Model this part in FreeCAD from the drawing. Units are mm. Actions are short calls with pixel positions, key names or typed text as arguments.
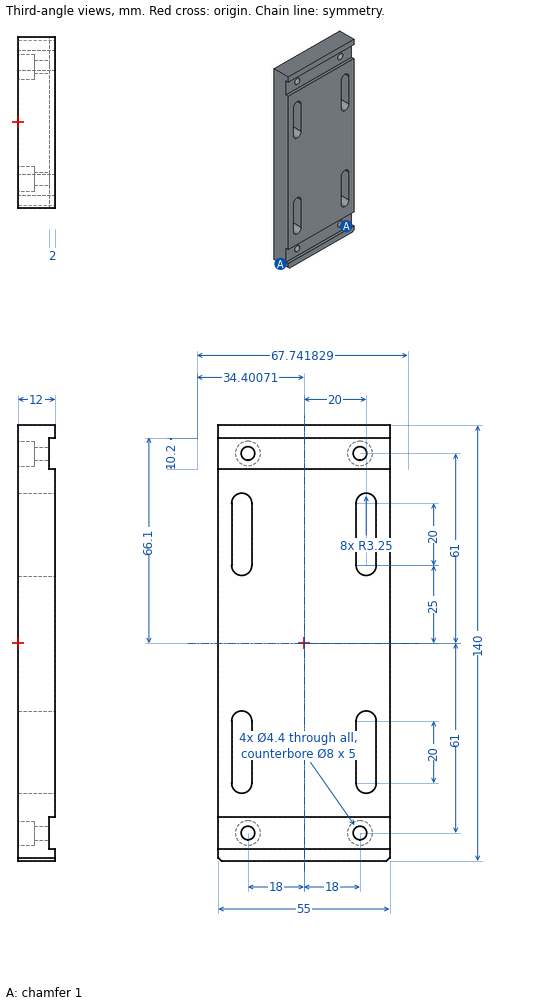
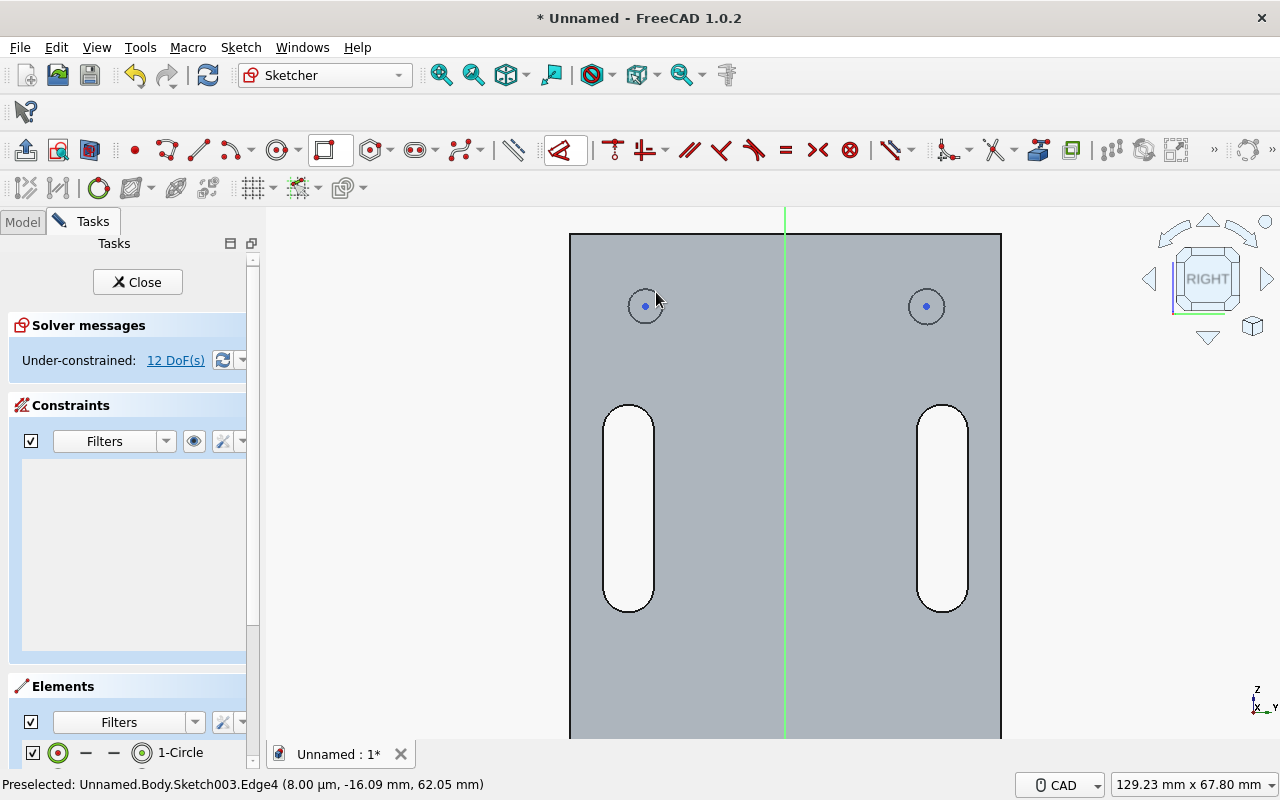
scroll(657, 292, down, 5)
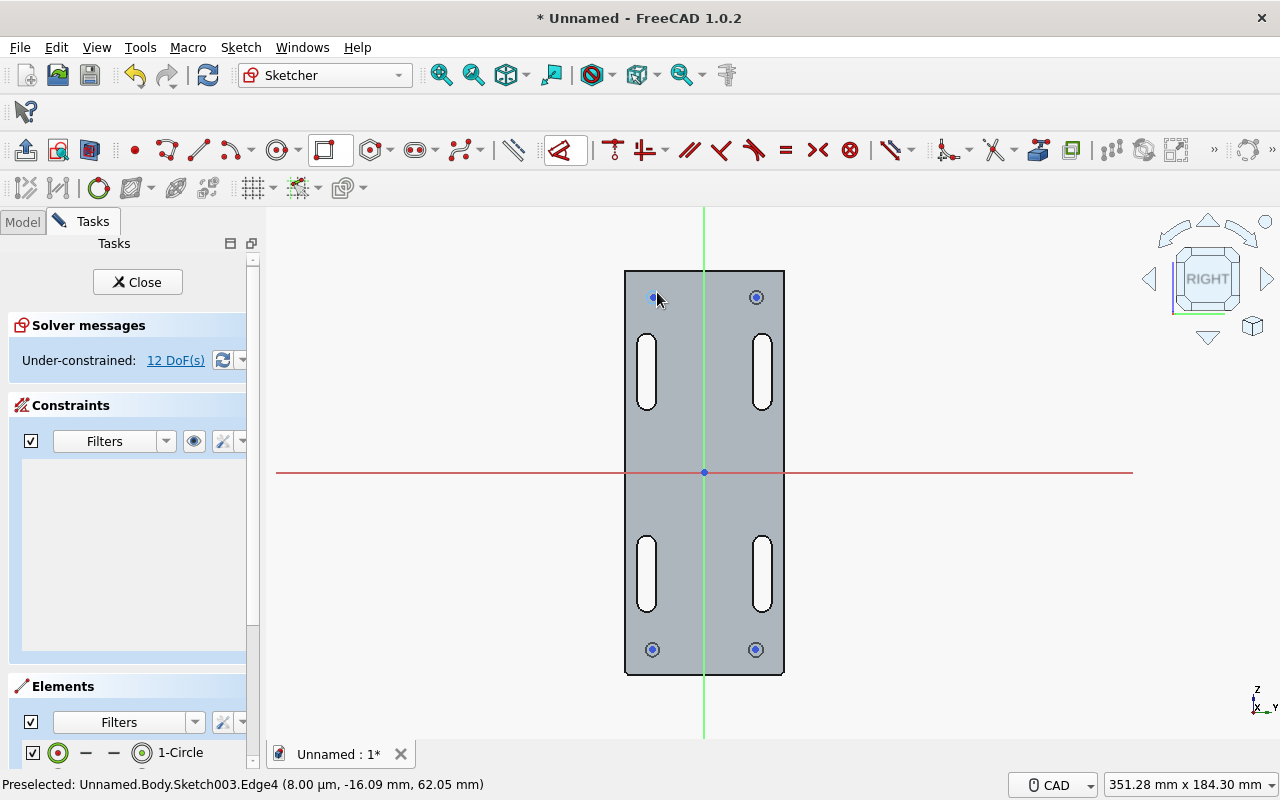
scroll(761, 645, up, 4)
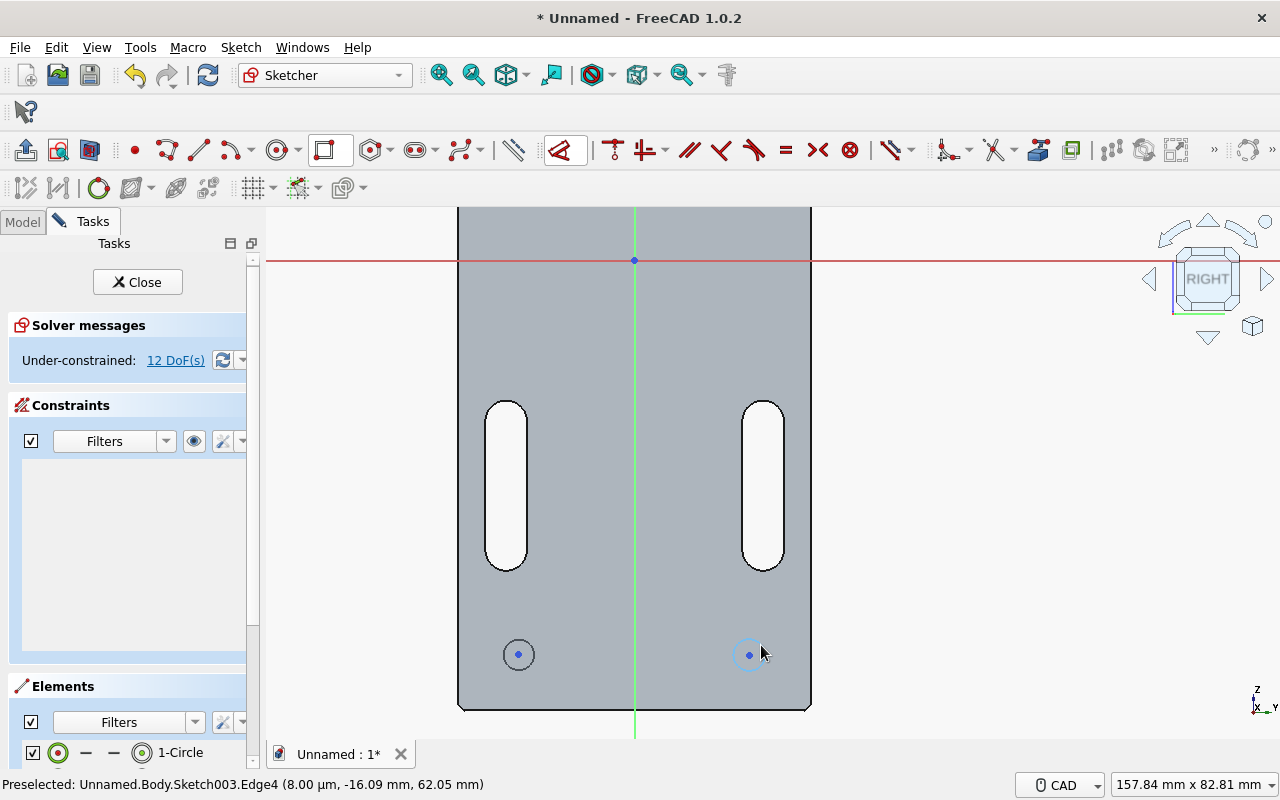
click(760, 644)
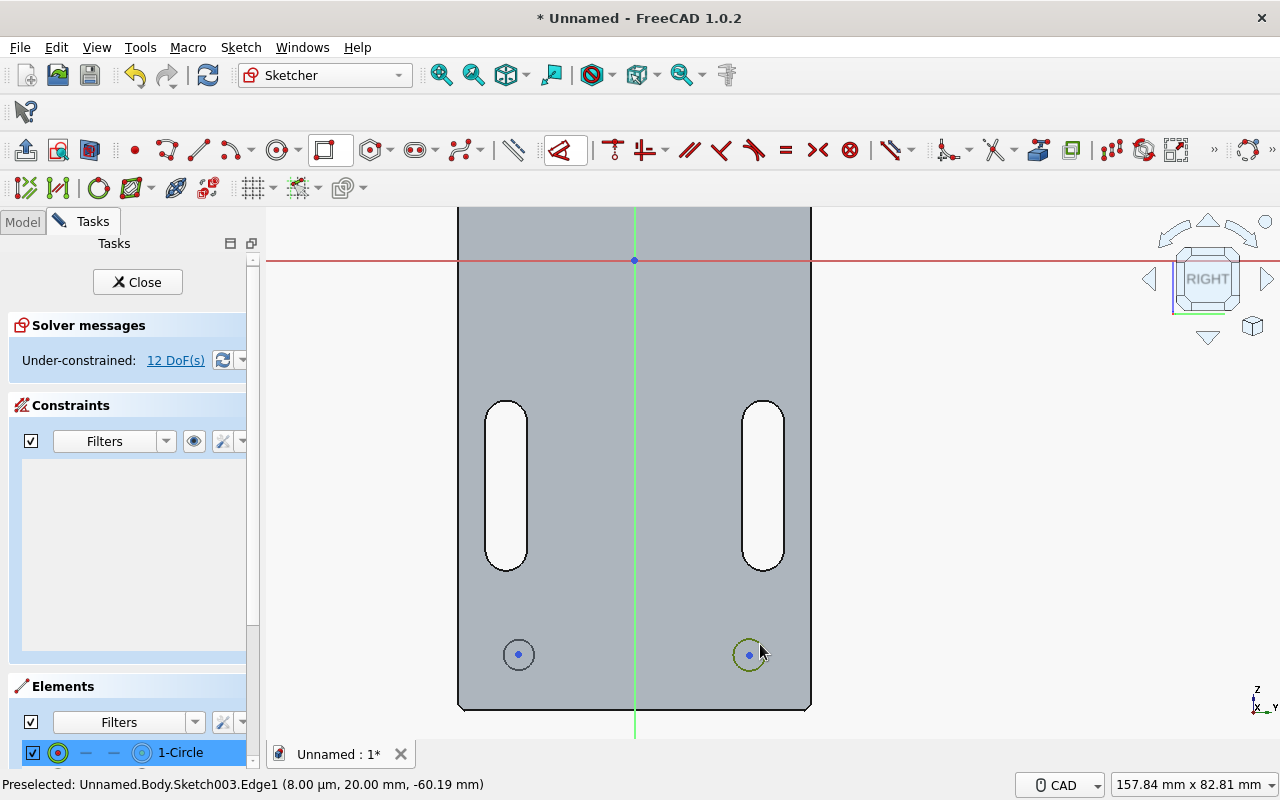
click(530, 644)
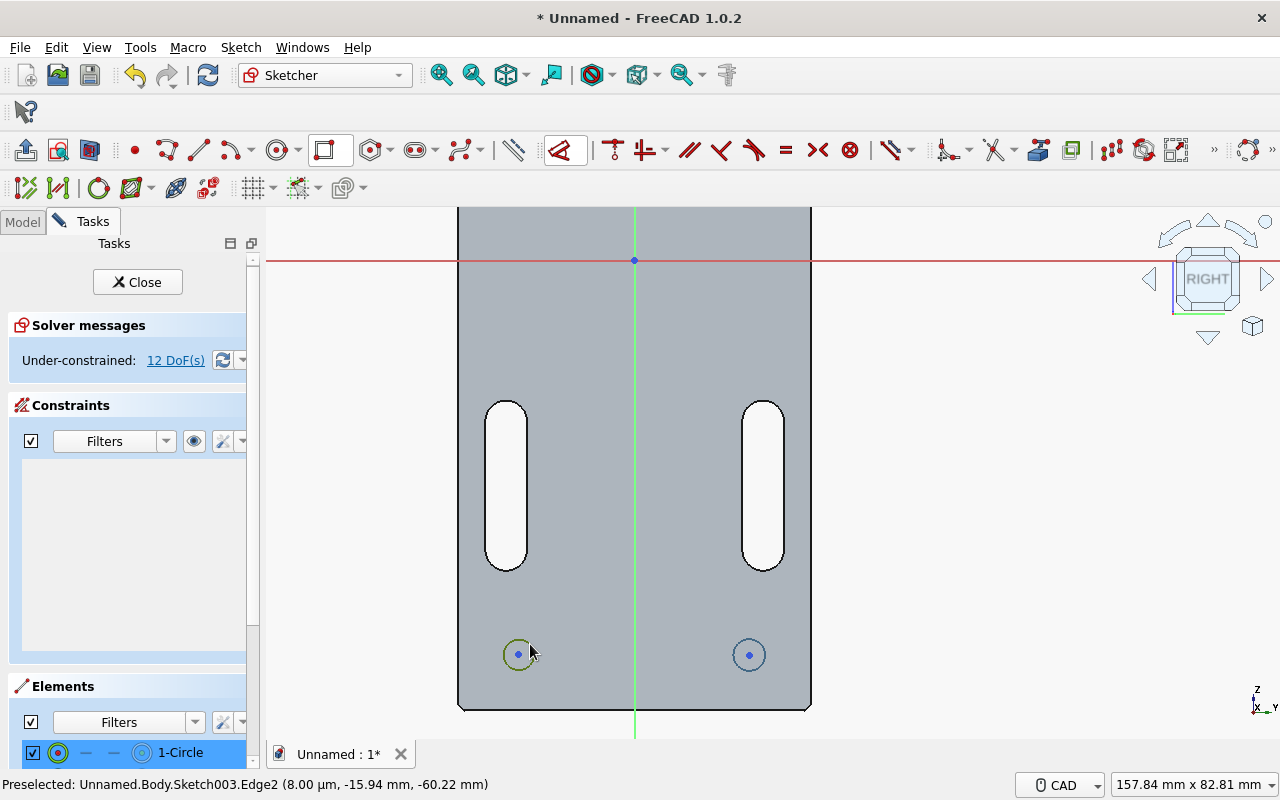
scroll(762, 646, down, 4)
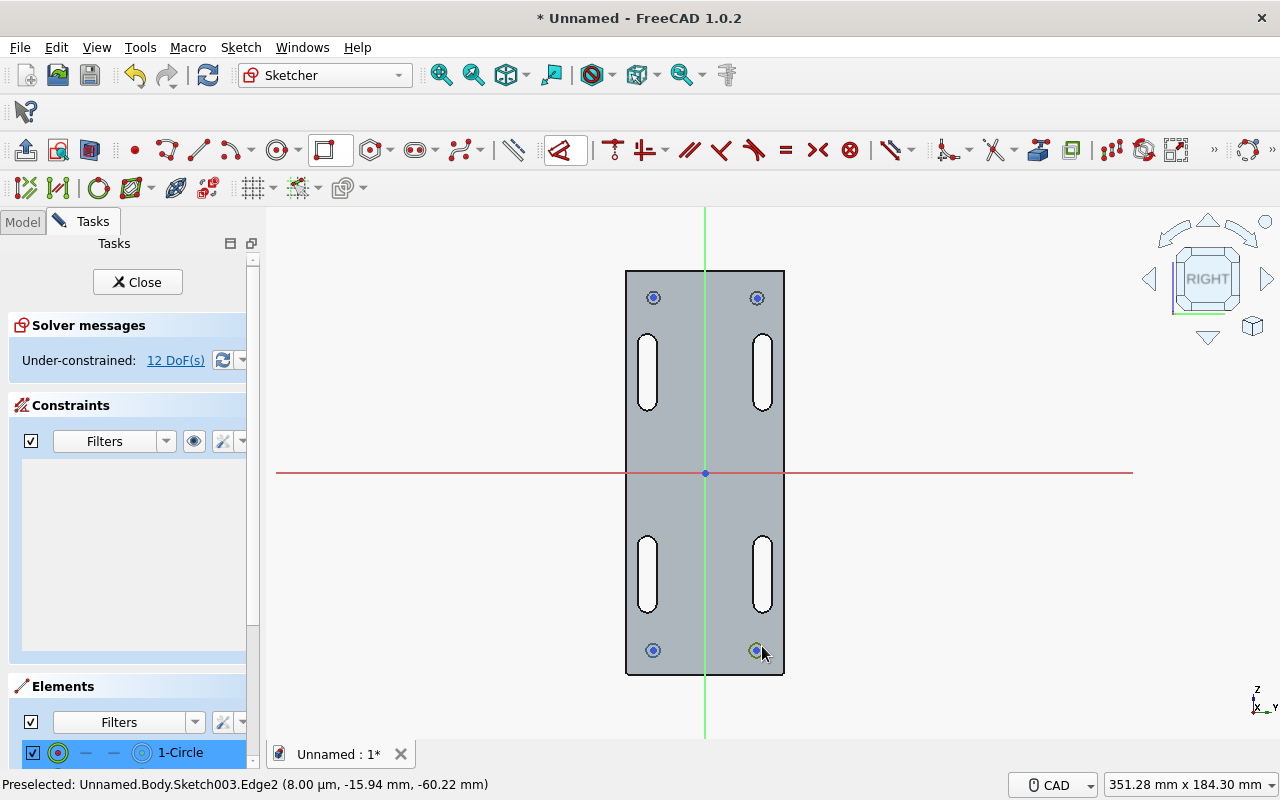
scroll(762, 293, up, 4)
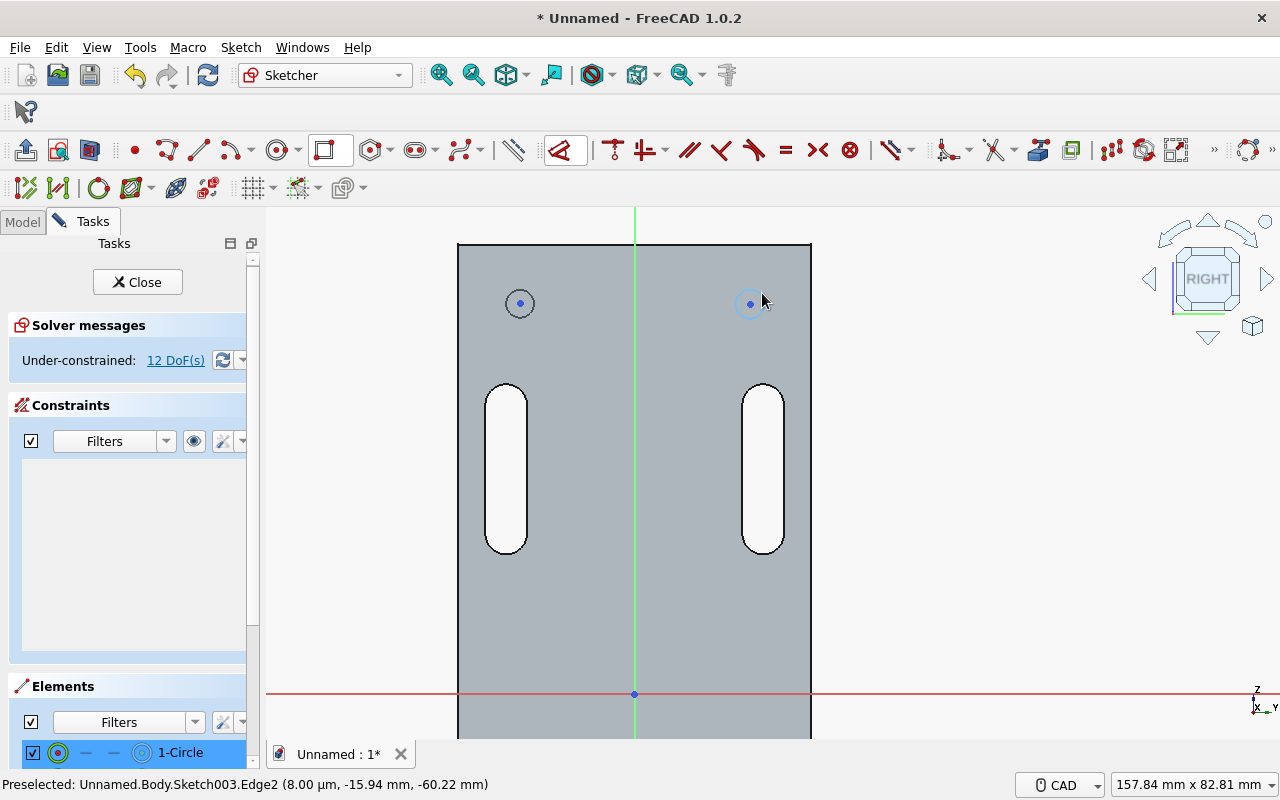
click(761, 294)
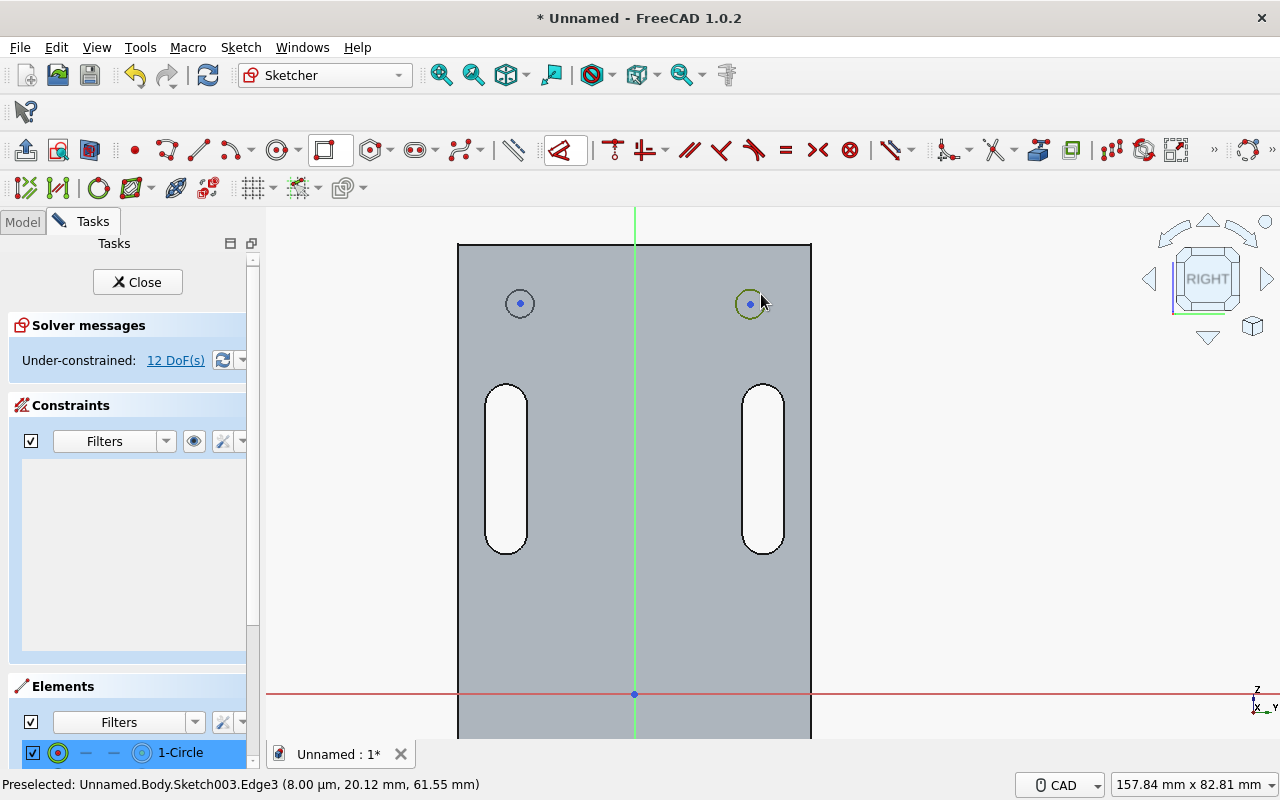
click(530, 294)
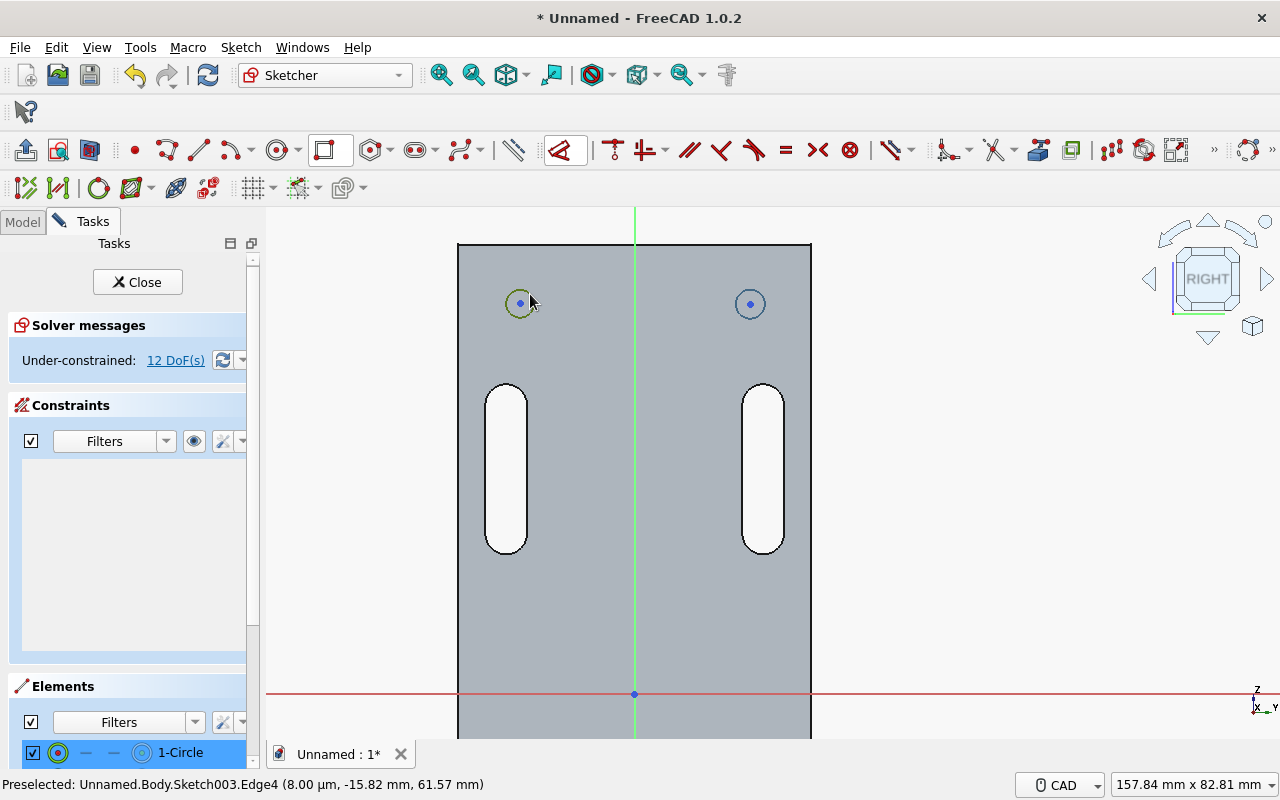
click(786, 150)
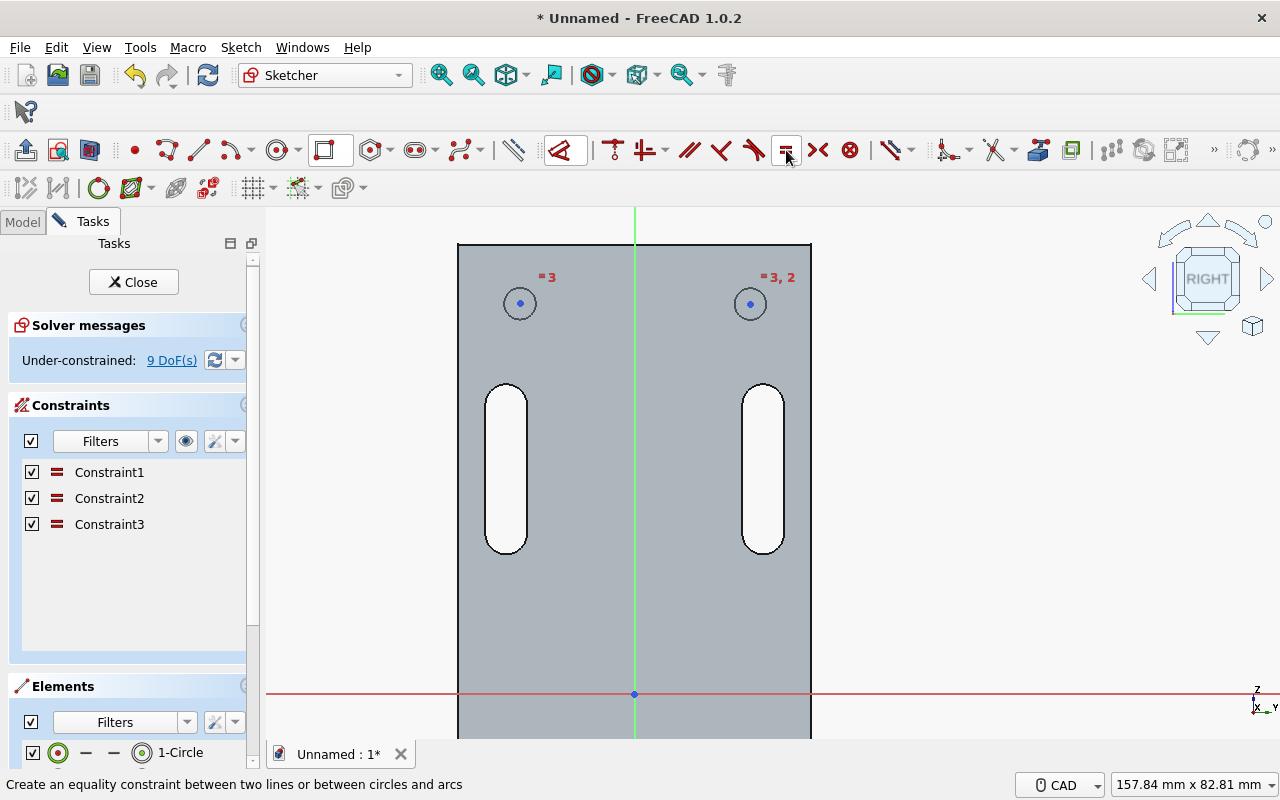
scroll(762, 293, down, 4)